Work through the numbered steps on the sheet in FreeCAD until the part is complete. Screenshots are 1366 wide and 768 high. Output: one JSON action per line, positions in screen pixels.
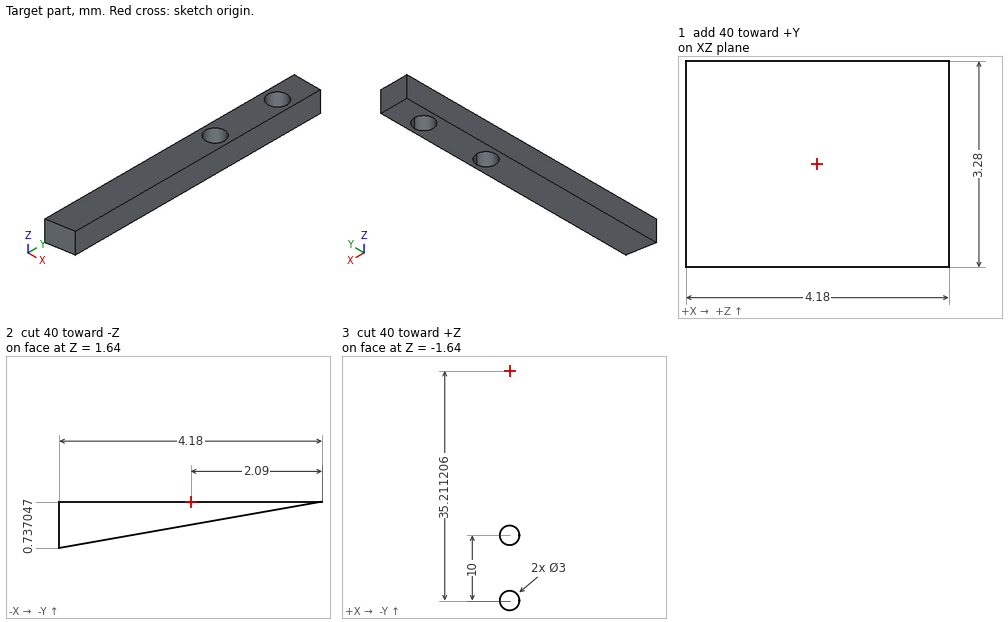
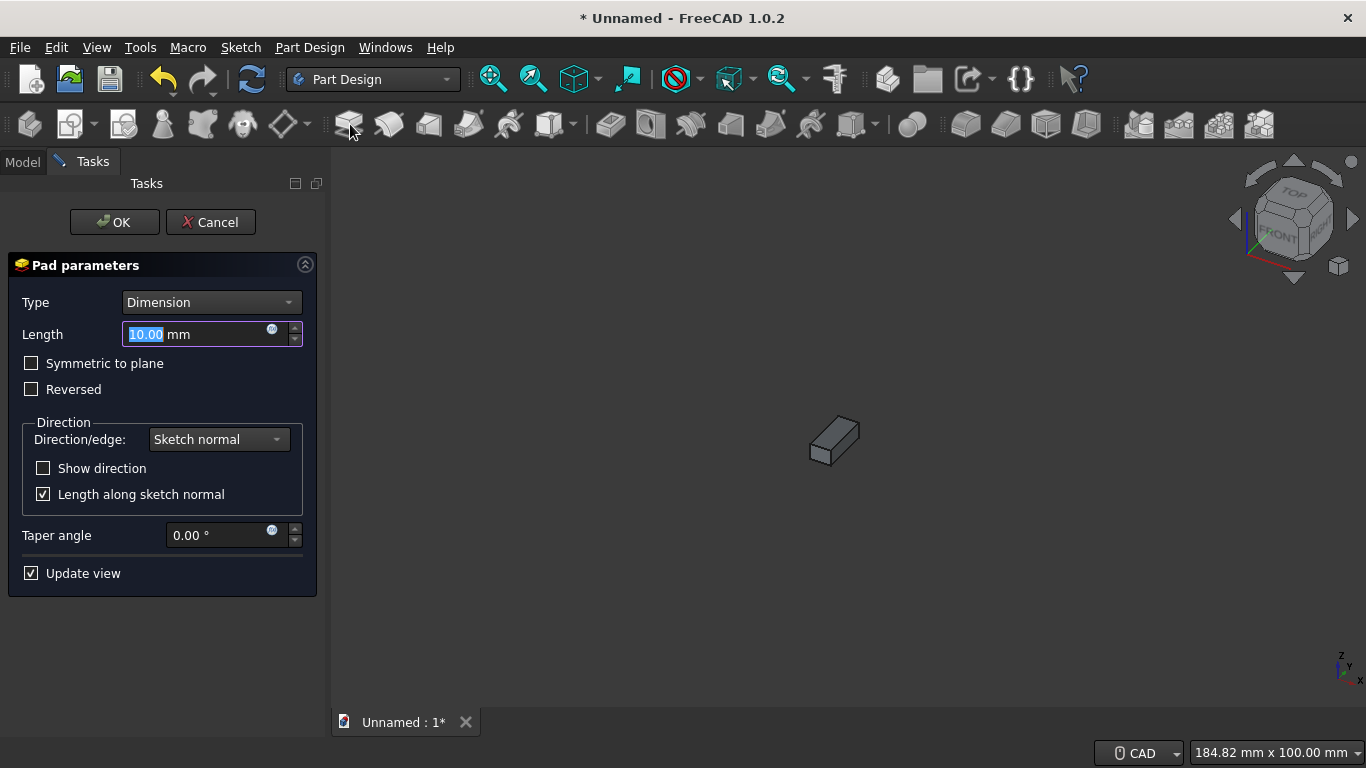
{"action": "type", "text": "40"}
{"action": "key", "text": "Tab"}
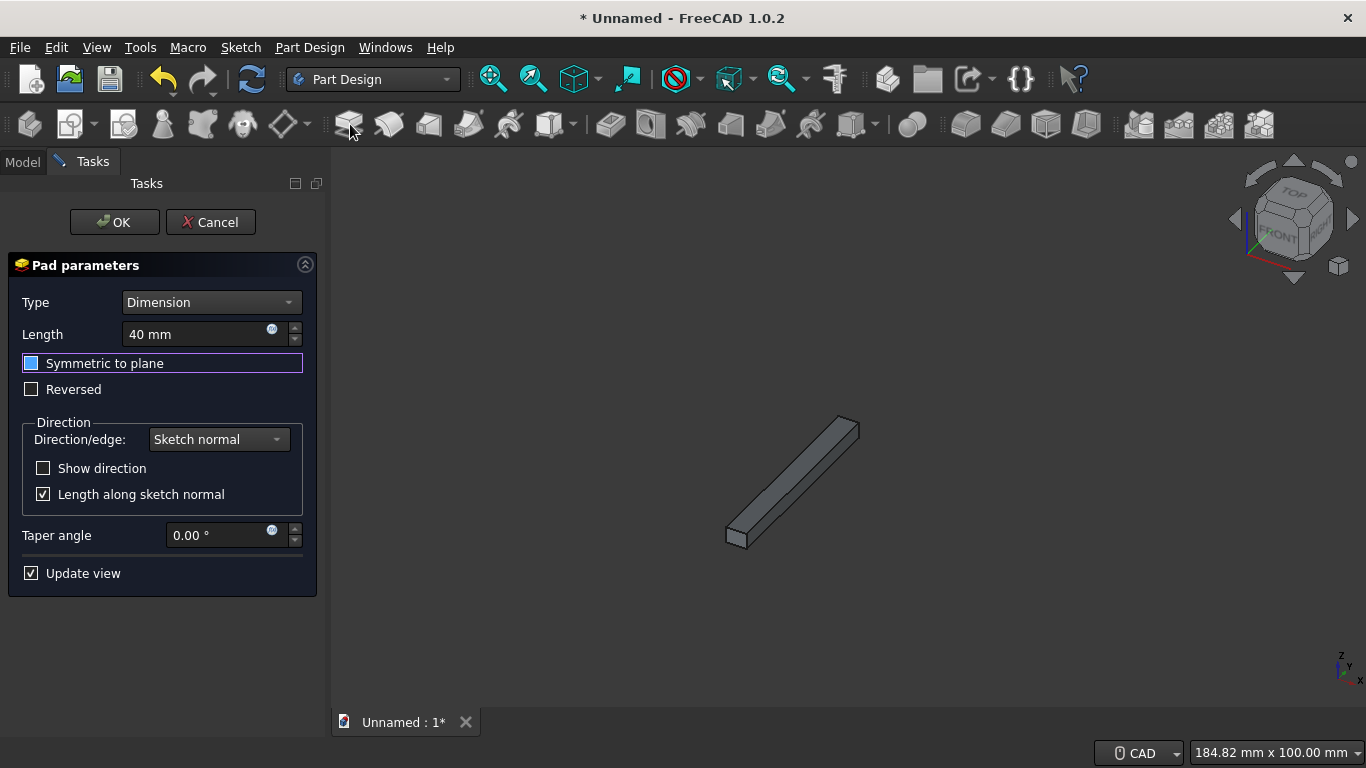
{"action": "left_click", "coordinate": [30, 389]}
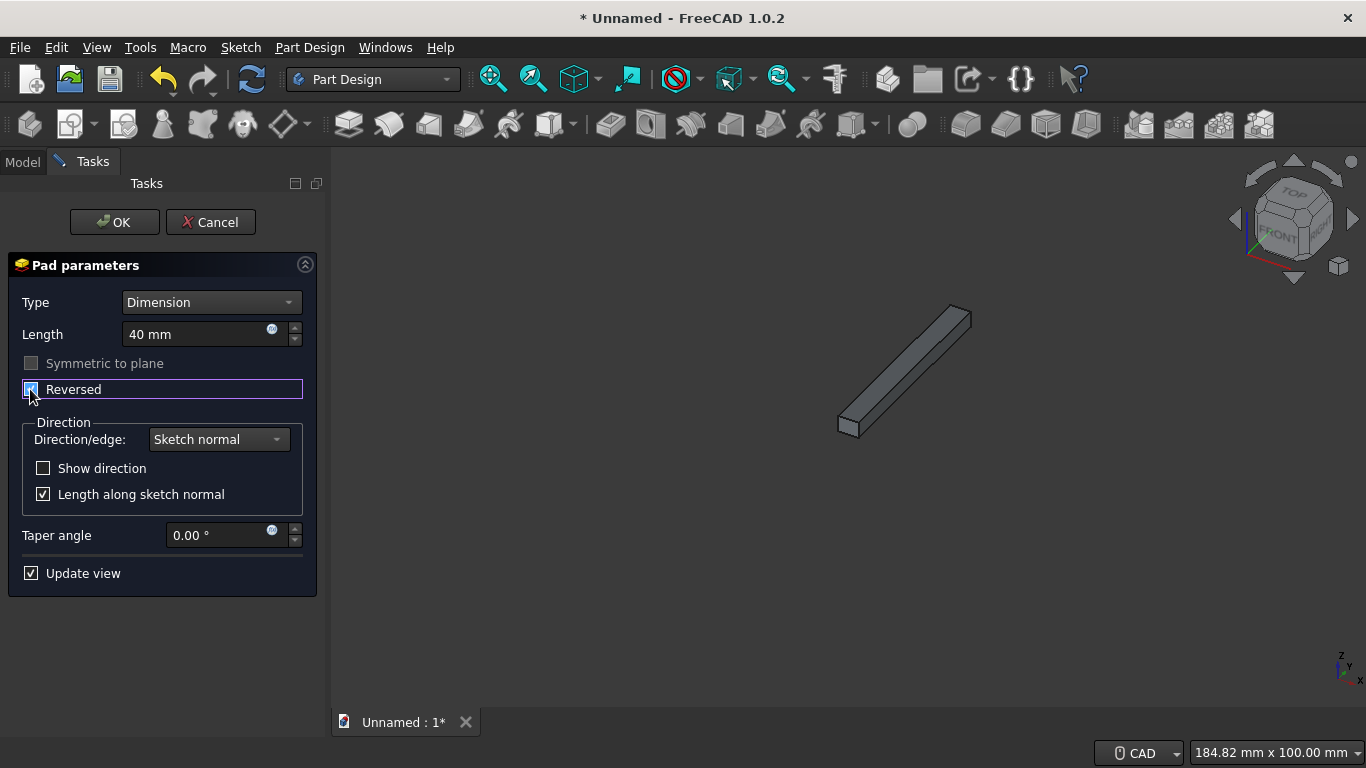
{"action": "left_click", "coordinate": [115, 222]}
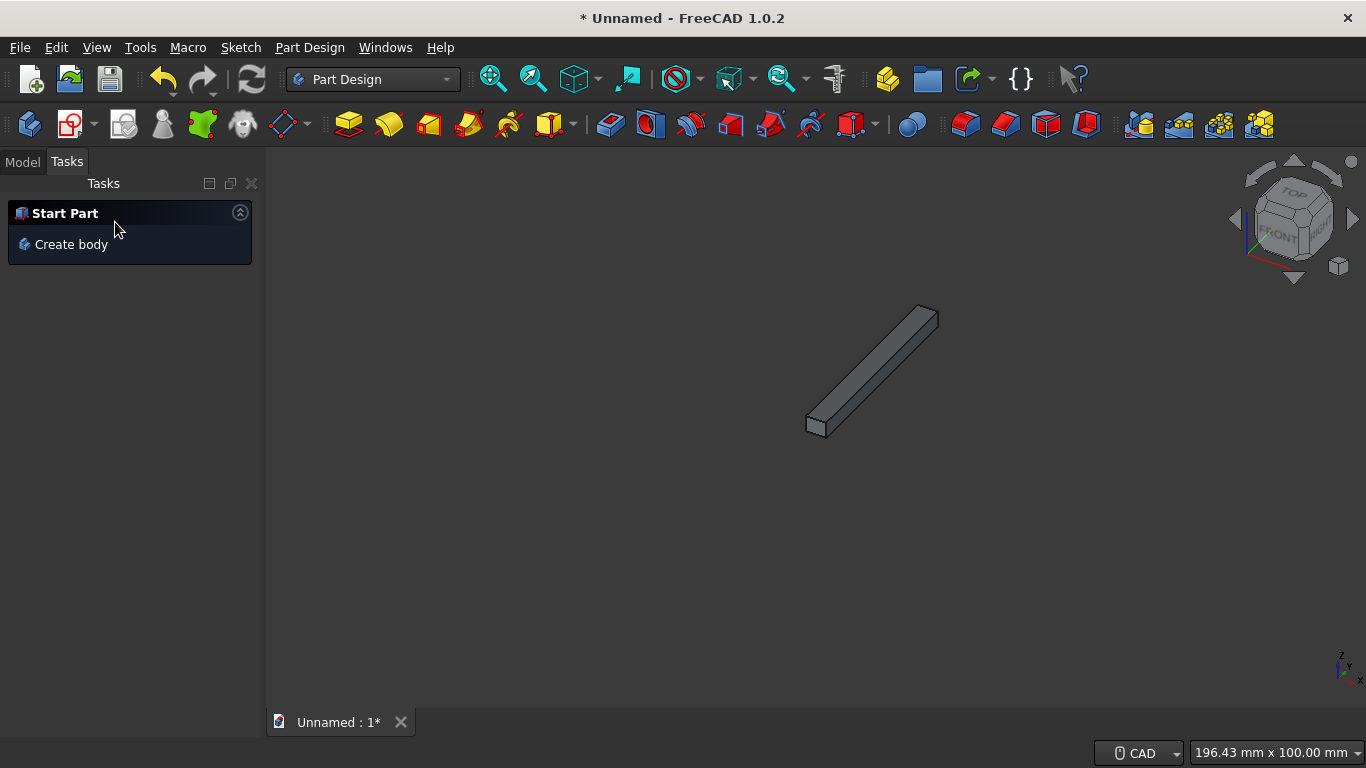
{"action": "left_click", "coordinate": [494, 80]}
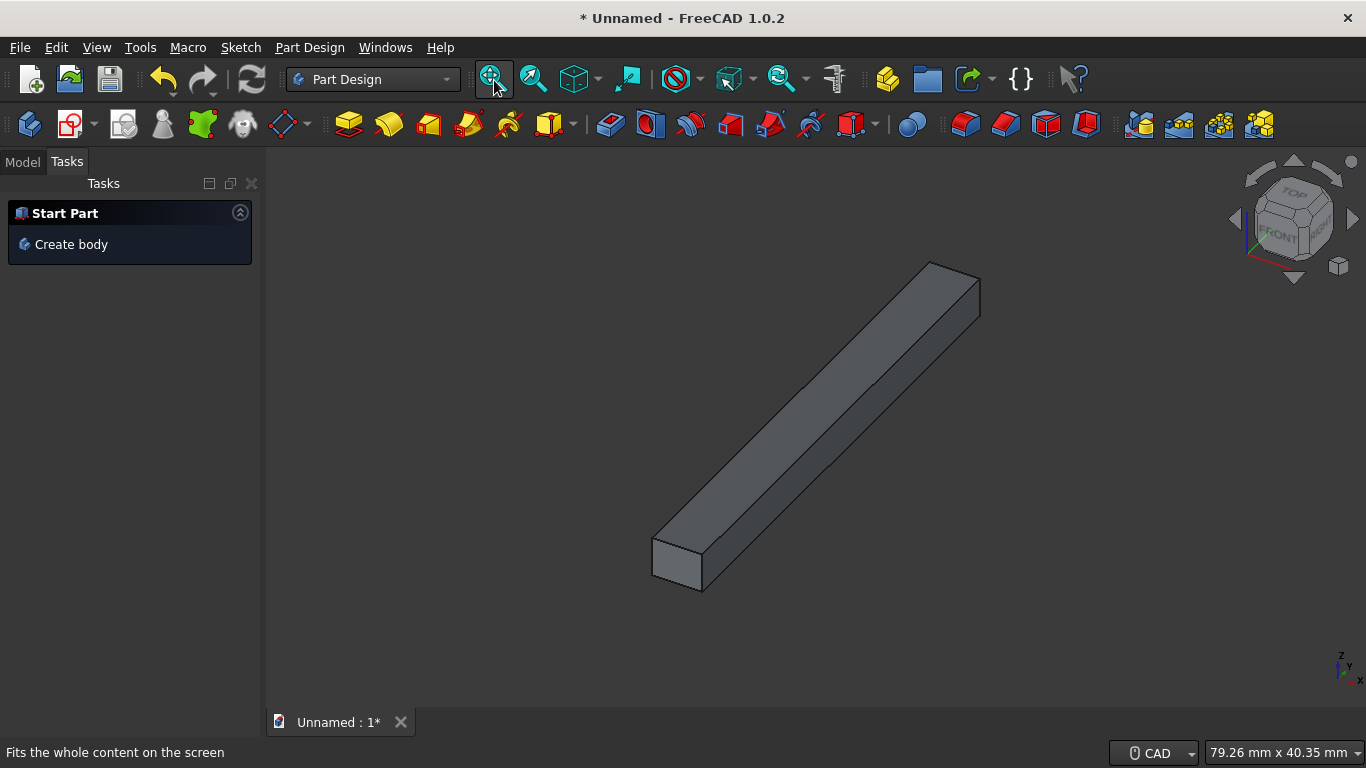
{"action": "left_click", "coordinate": [935, 289]}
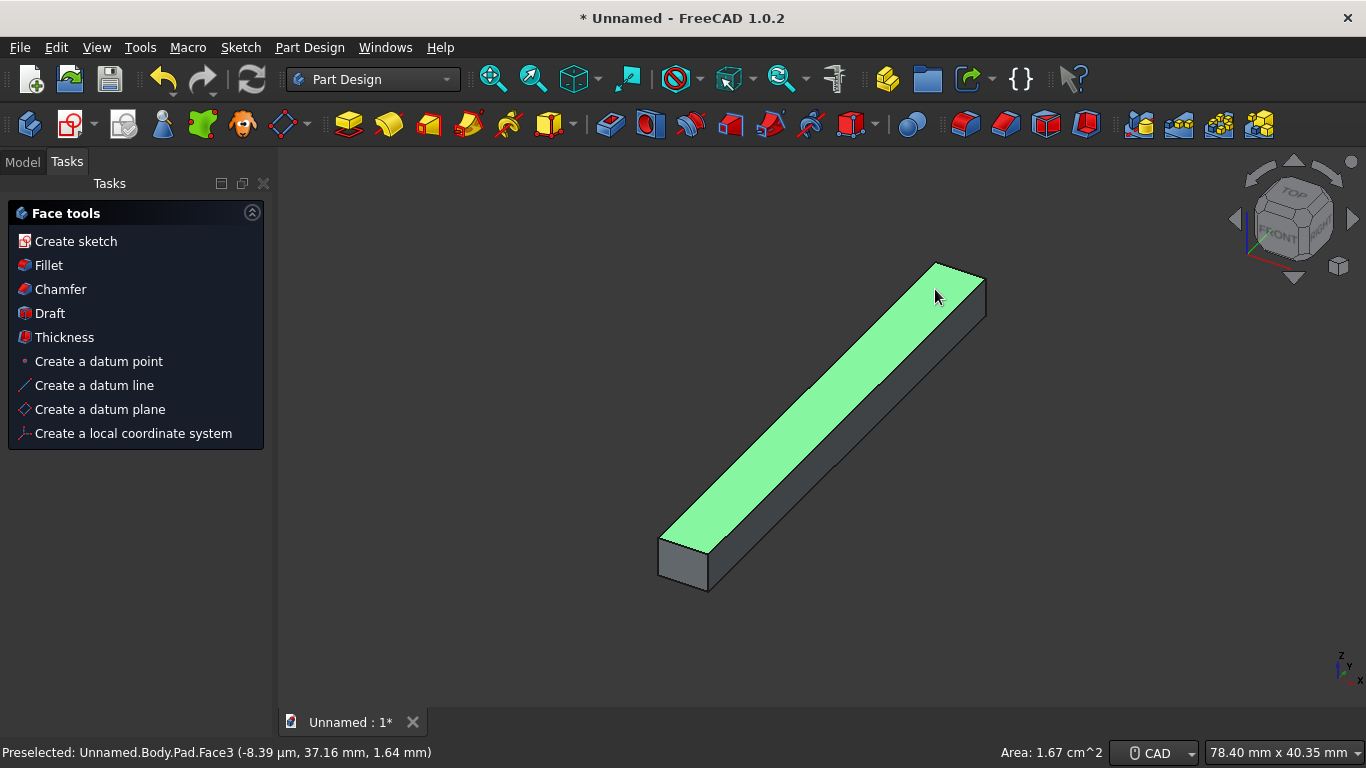
{"action": "left_click", "coordinate": [70, 124]}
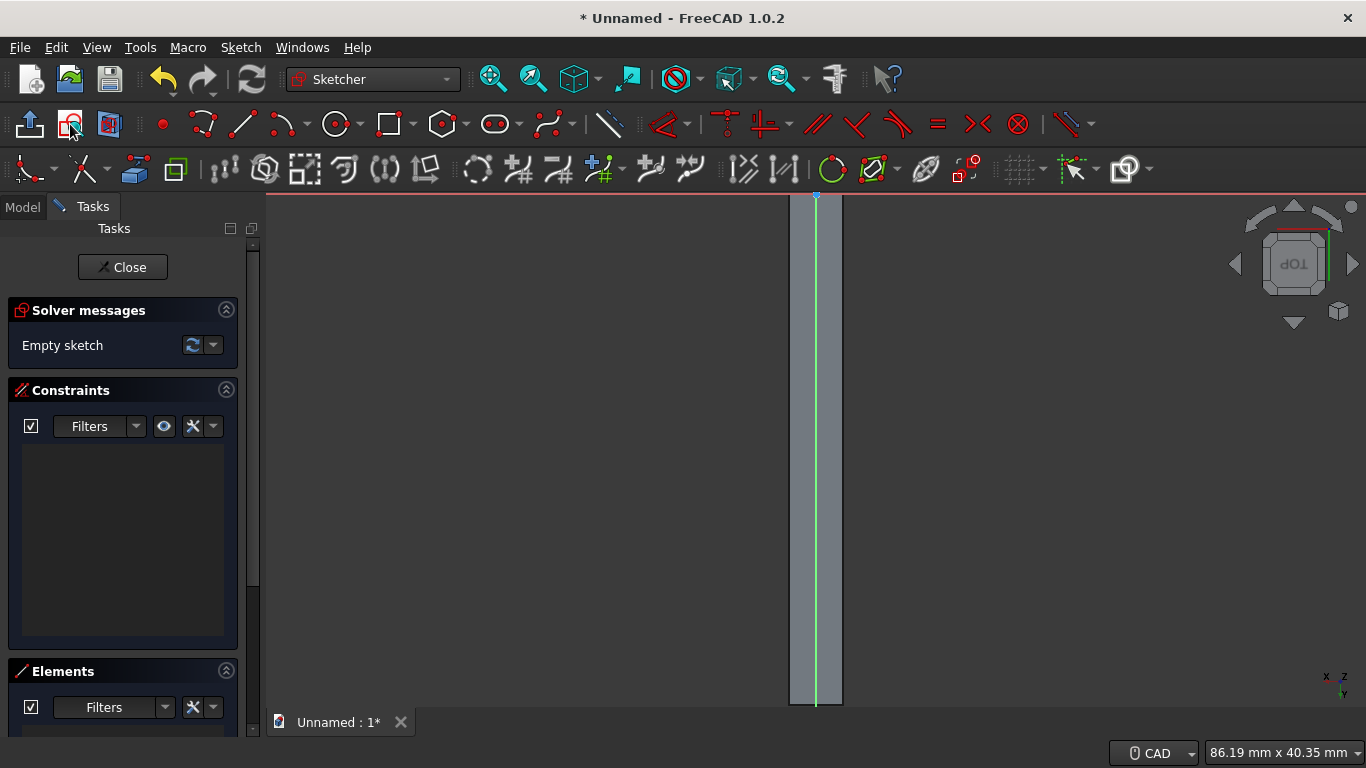
{"action": "scroll", "coordinate": [748, 450], "scroll_direction": "down", "scroll_amount": 5}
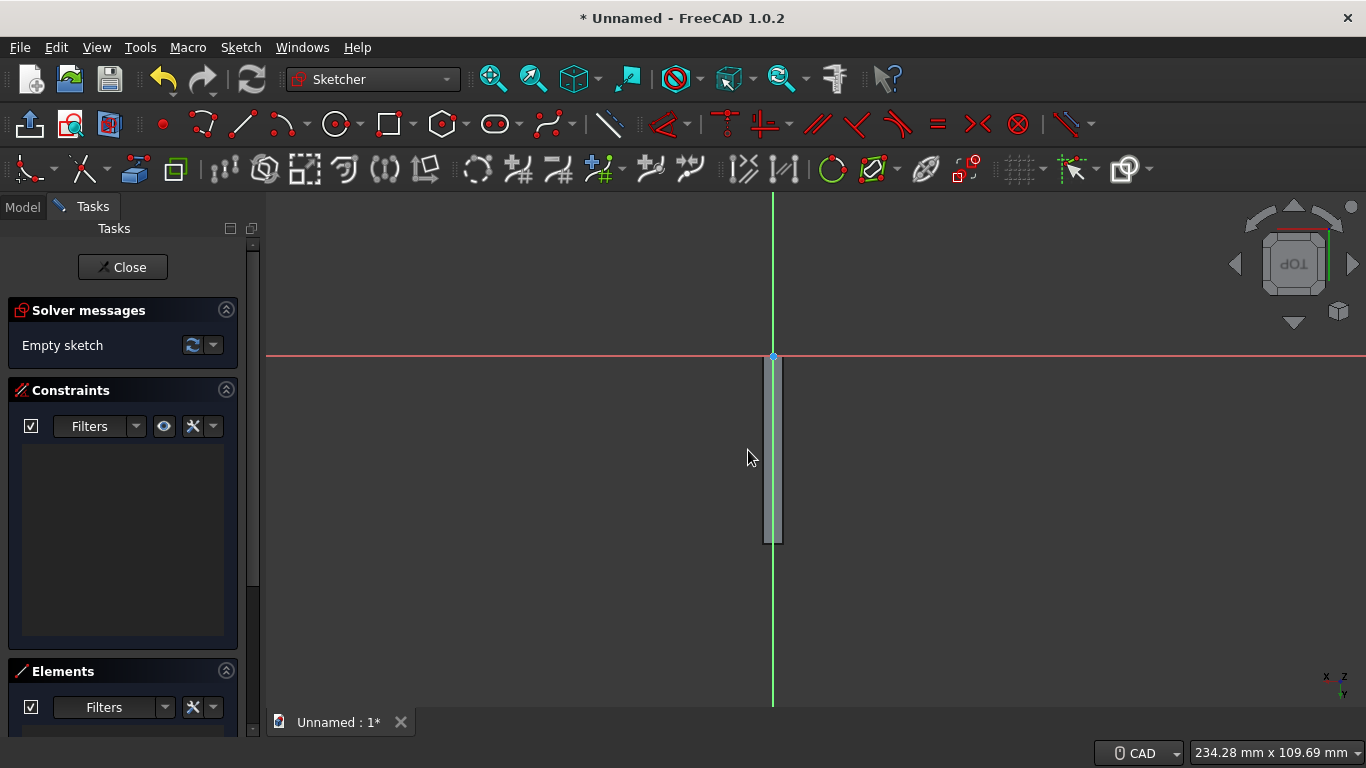
{"action": "scroll", "coordinate": [775, 353], "scroll_direction": "up", "scroll_amount": 15}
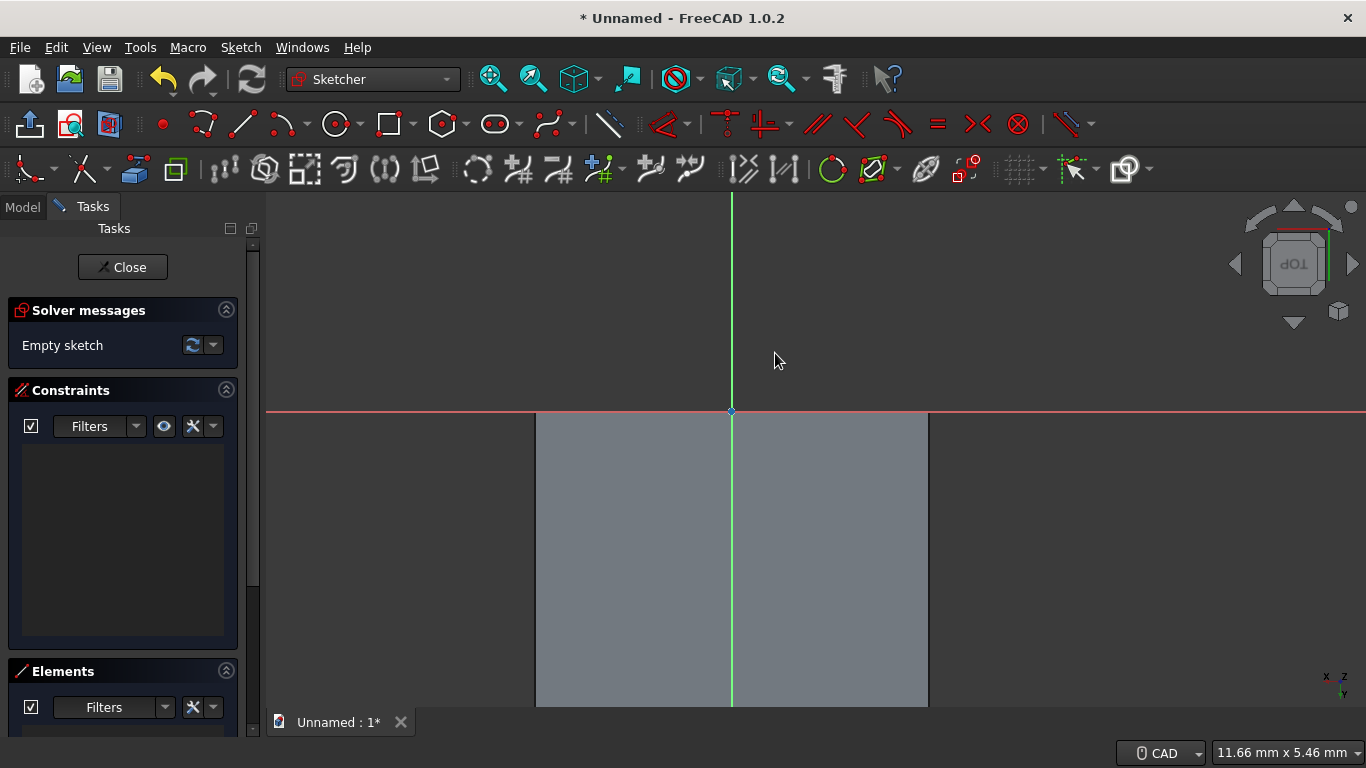
{"action": "scroll", "coordinate": [700, 441], "scroll_direction": "up", "scroll_amount": 2}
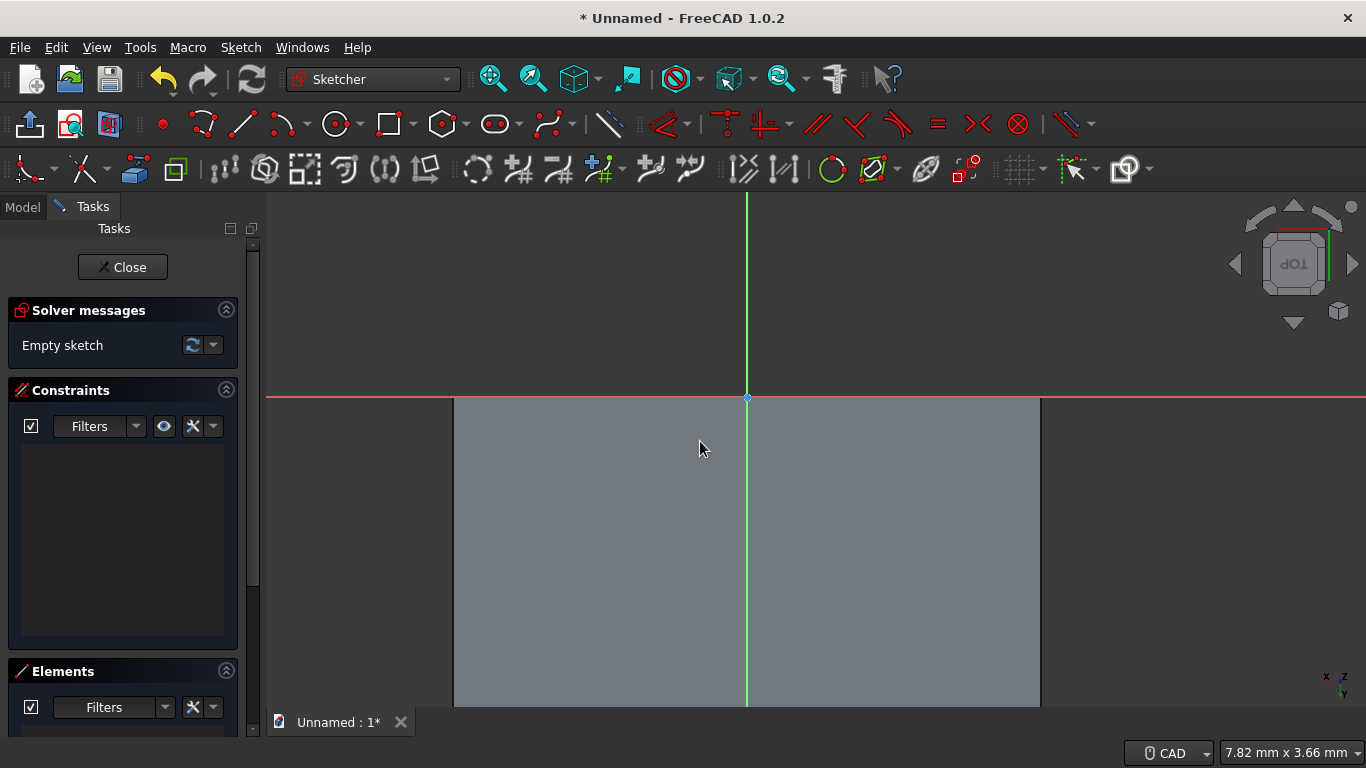
{"action": "left_click", "coordinate": [204, 124]}